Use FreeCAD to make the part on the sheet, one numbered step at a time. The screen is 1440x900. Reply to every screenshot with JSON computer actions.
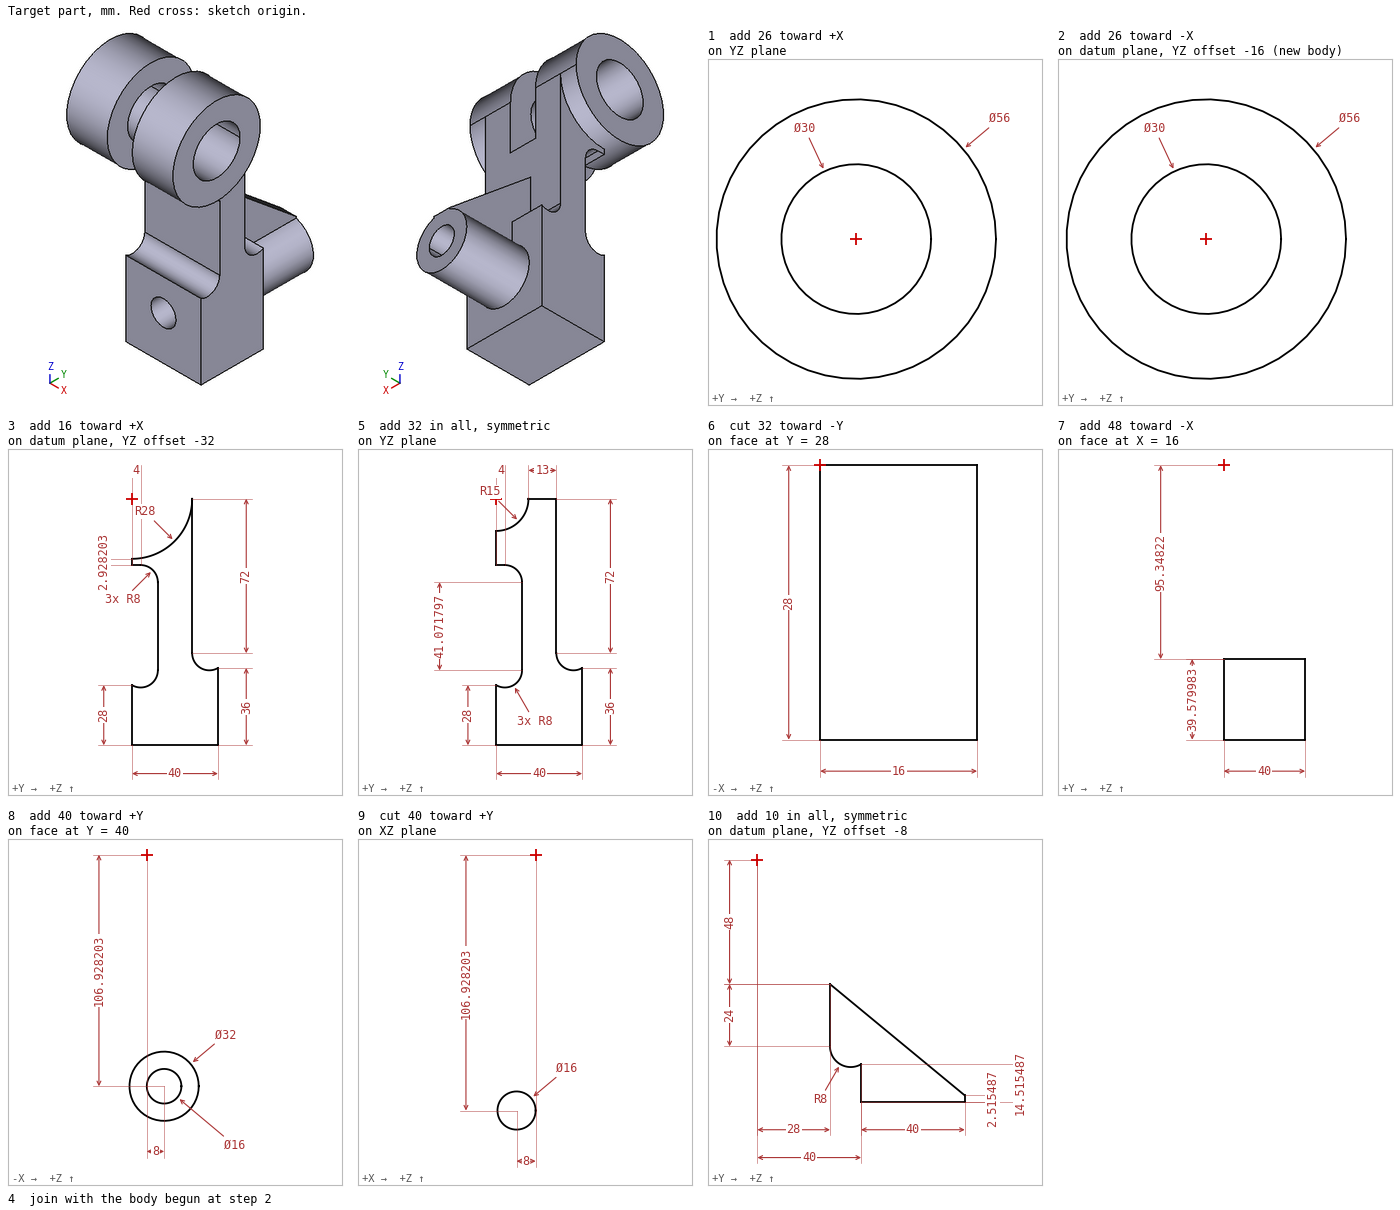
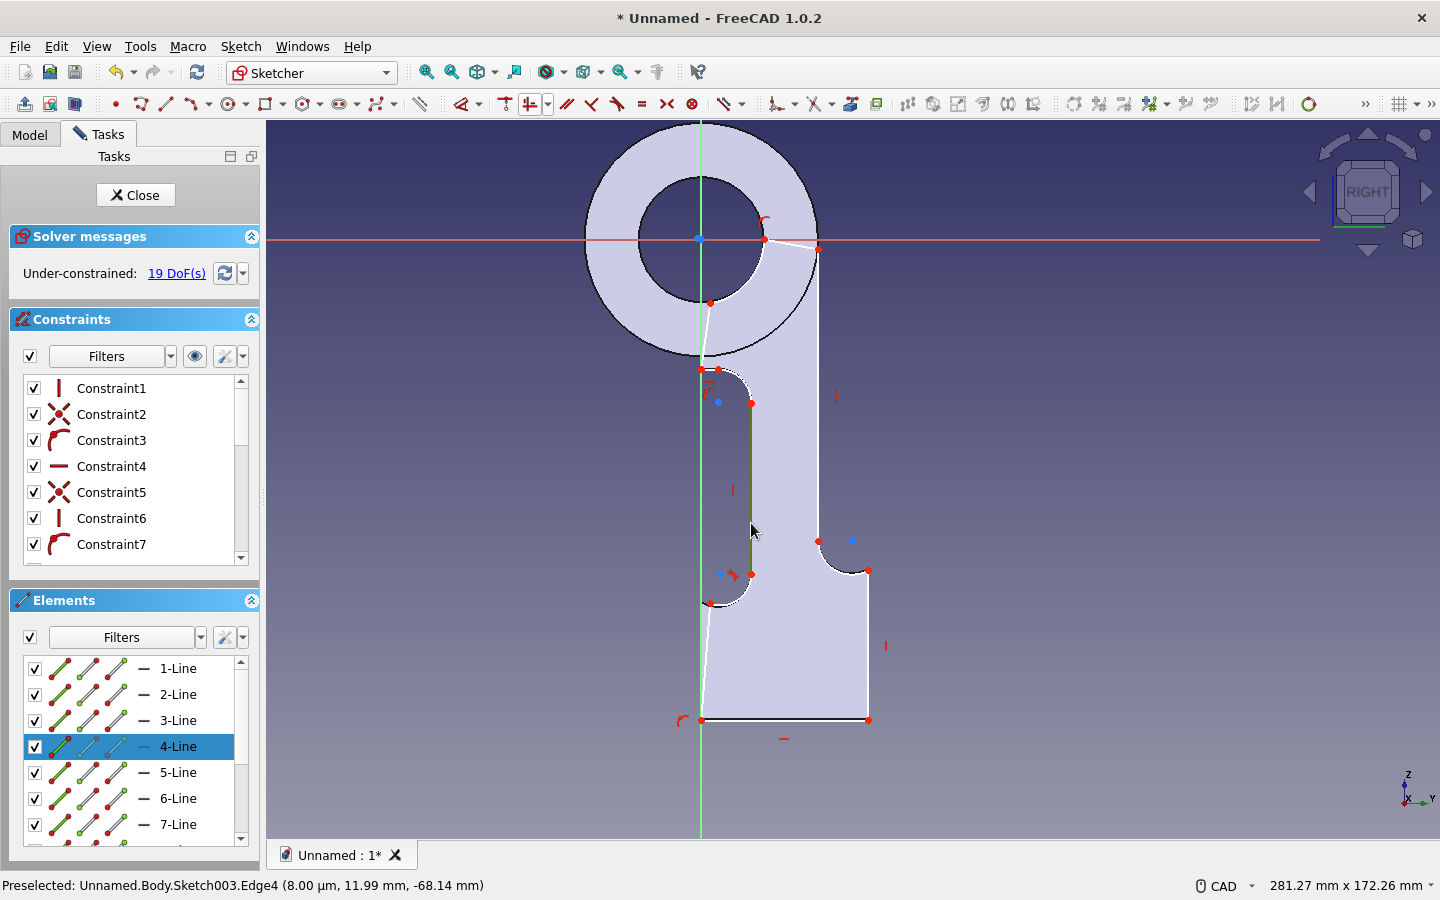
{"action": "left_click", "coordinate": [748, 388]}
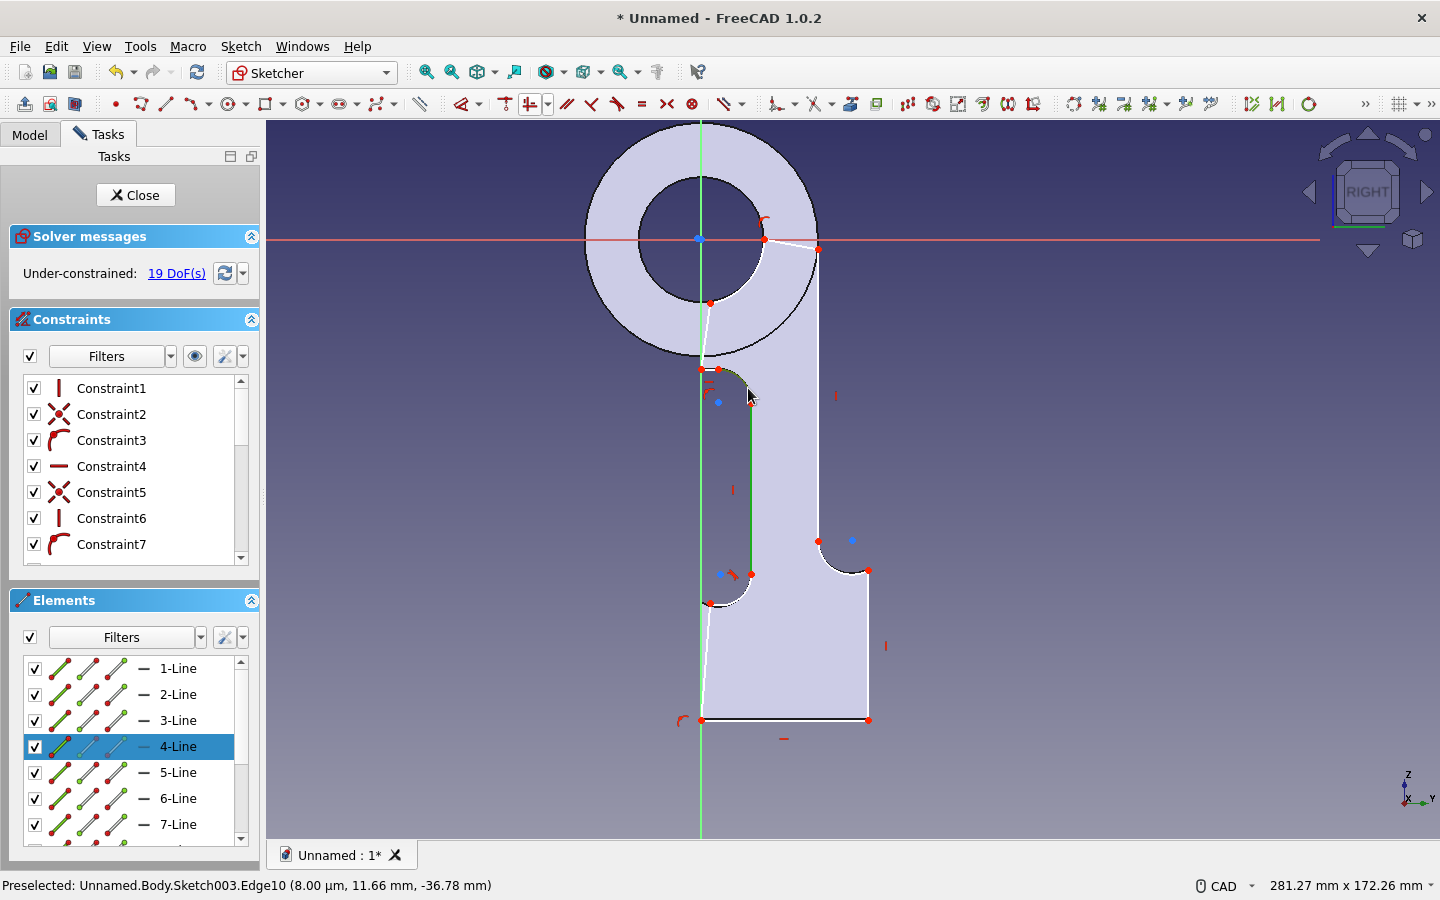
{"action": "key", "text": "t"}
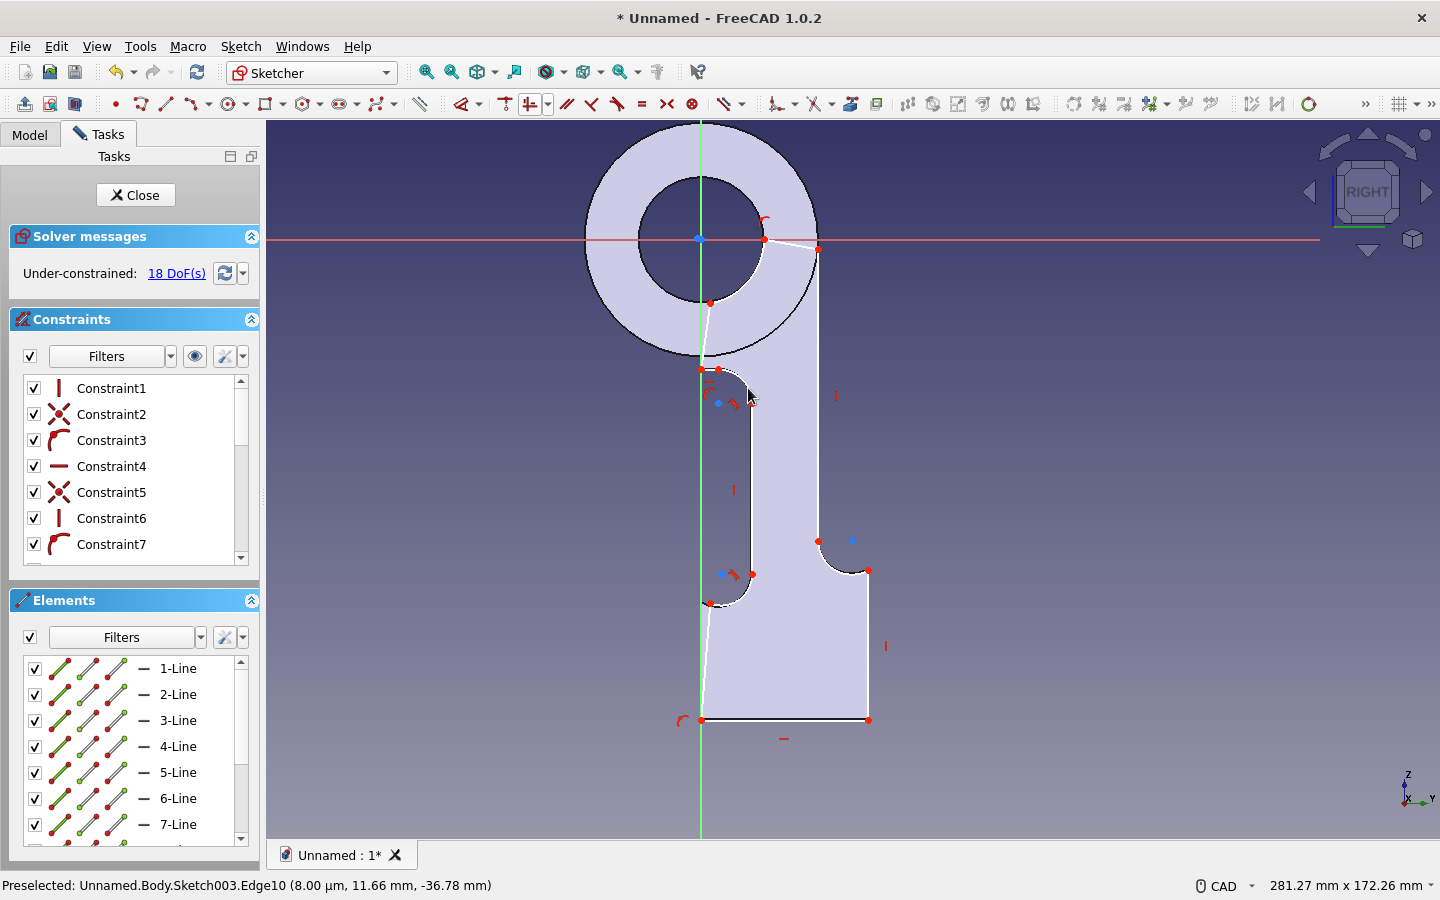
{"action": "scroll", "coordinate": [710, 370], "scroll_direction": "up", "scroll_amount": 3}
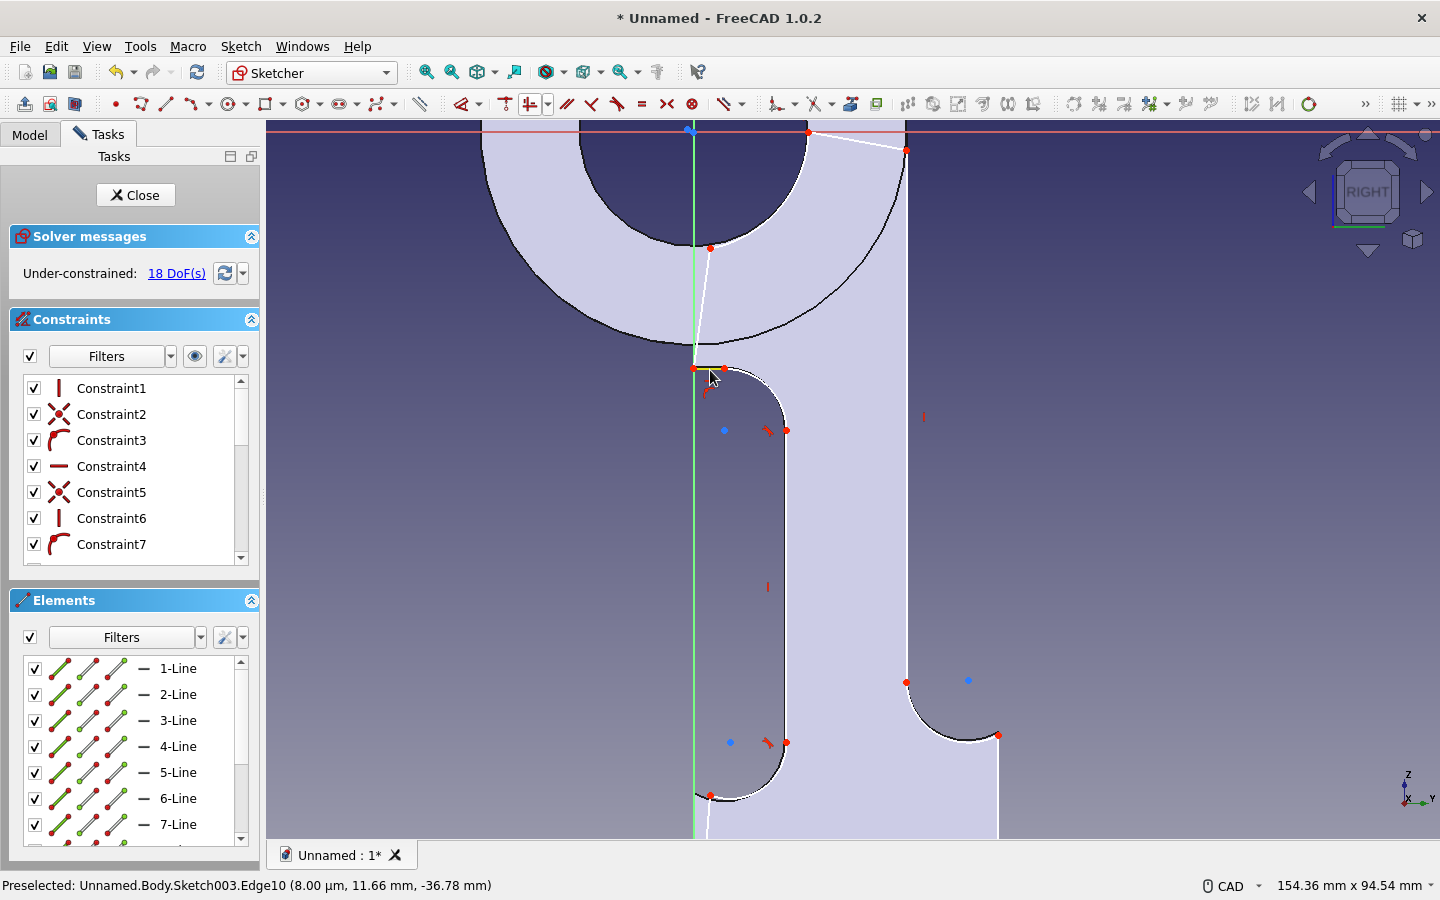
{"action": "left_click", "coordinate": [709, 369]}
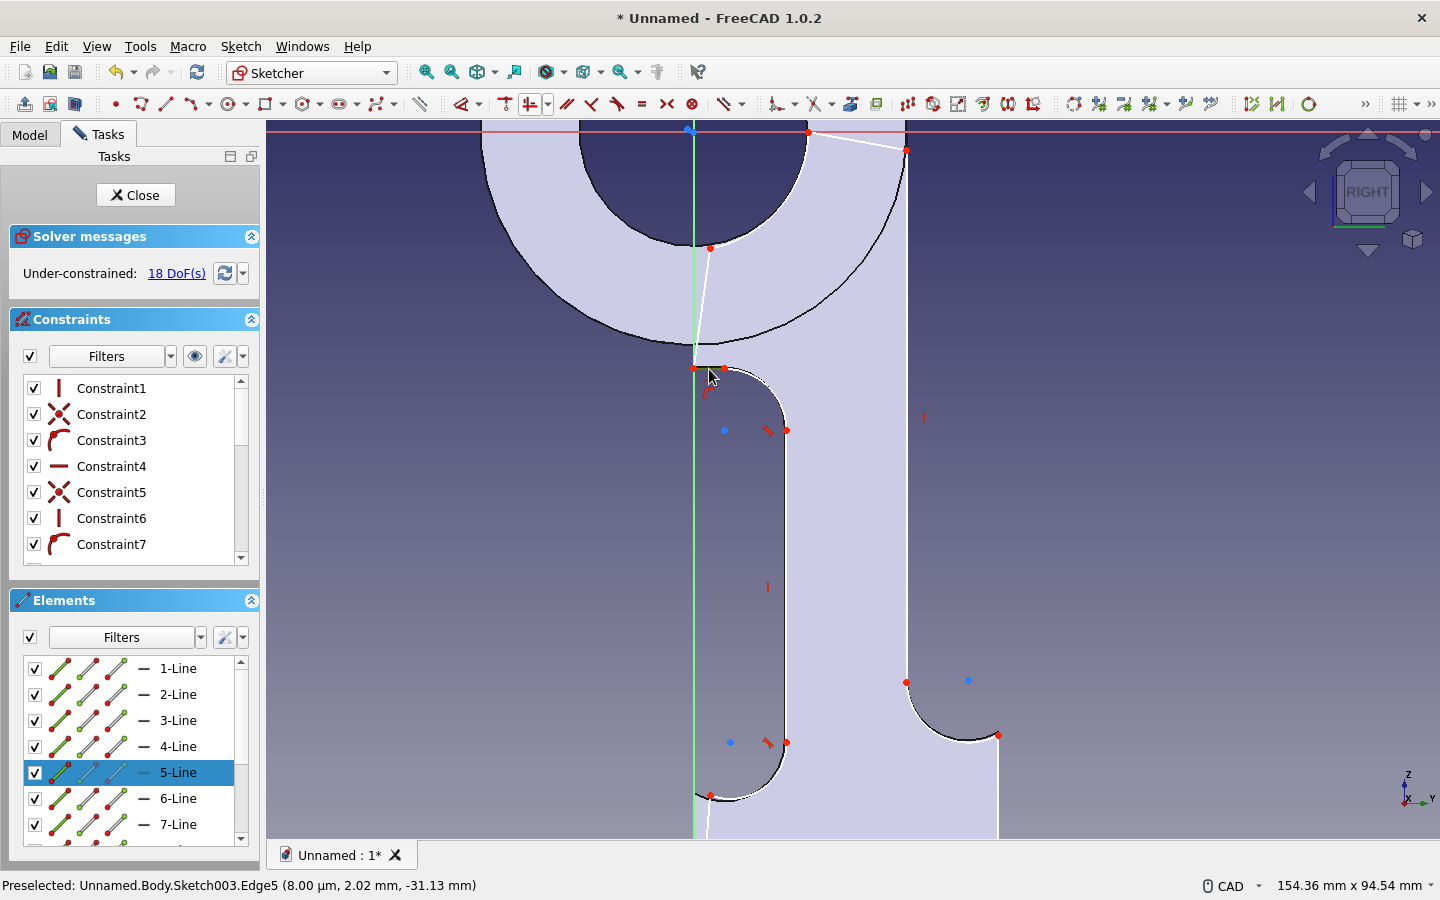
{"action": "left_click", "coordinate": [780, 403]}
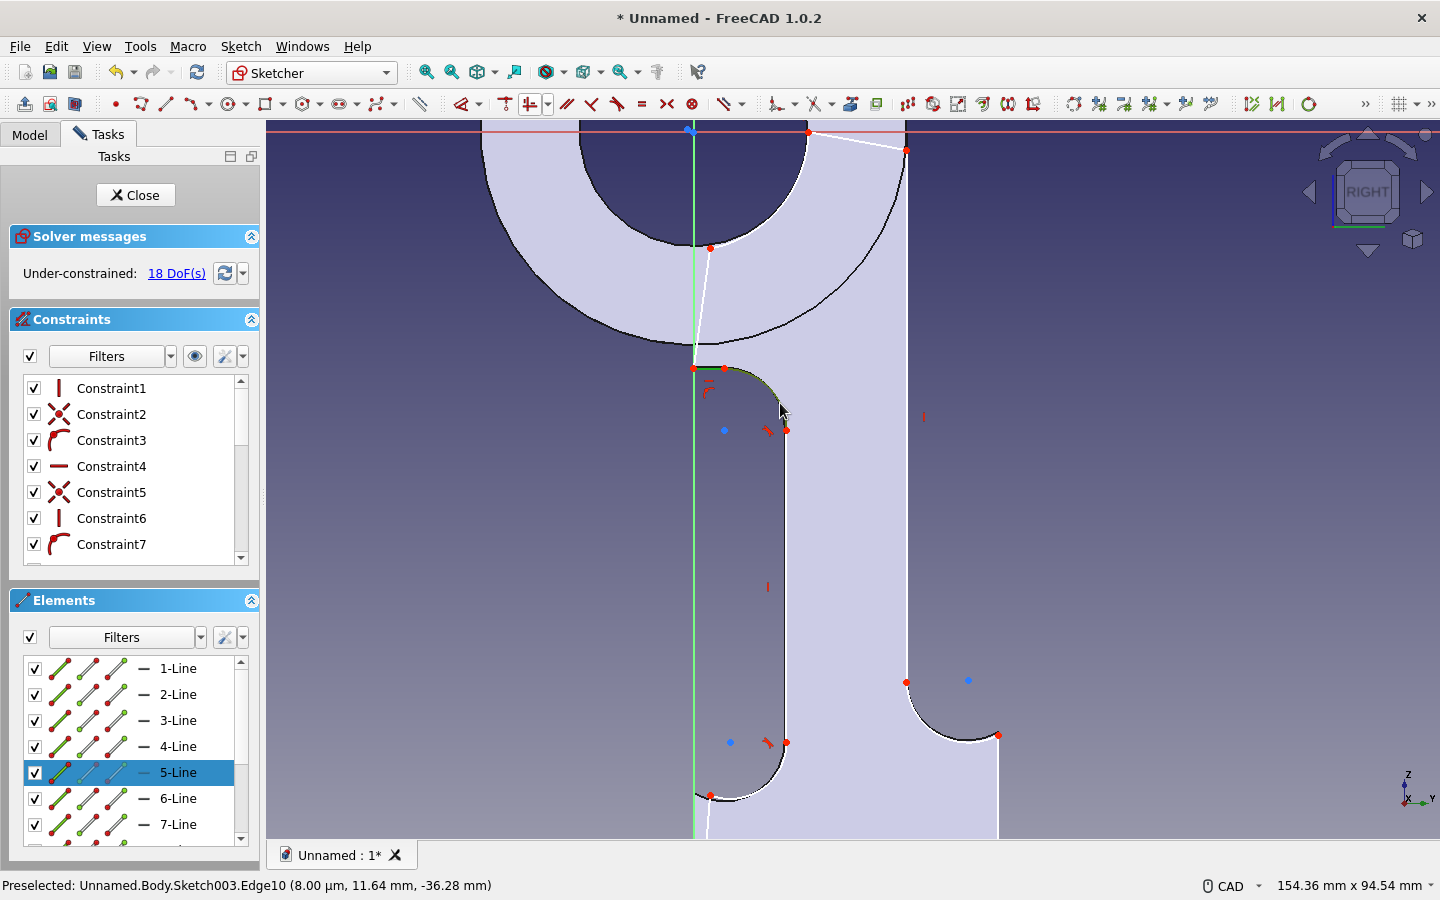
{"action": "key", "text": "t"}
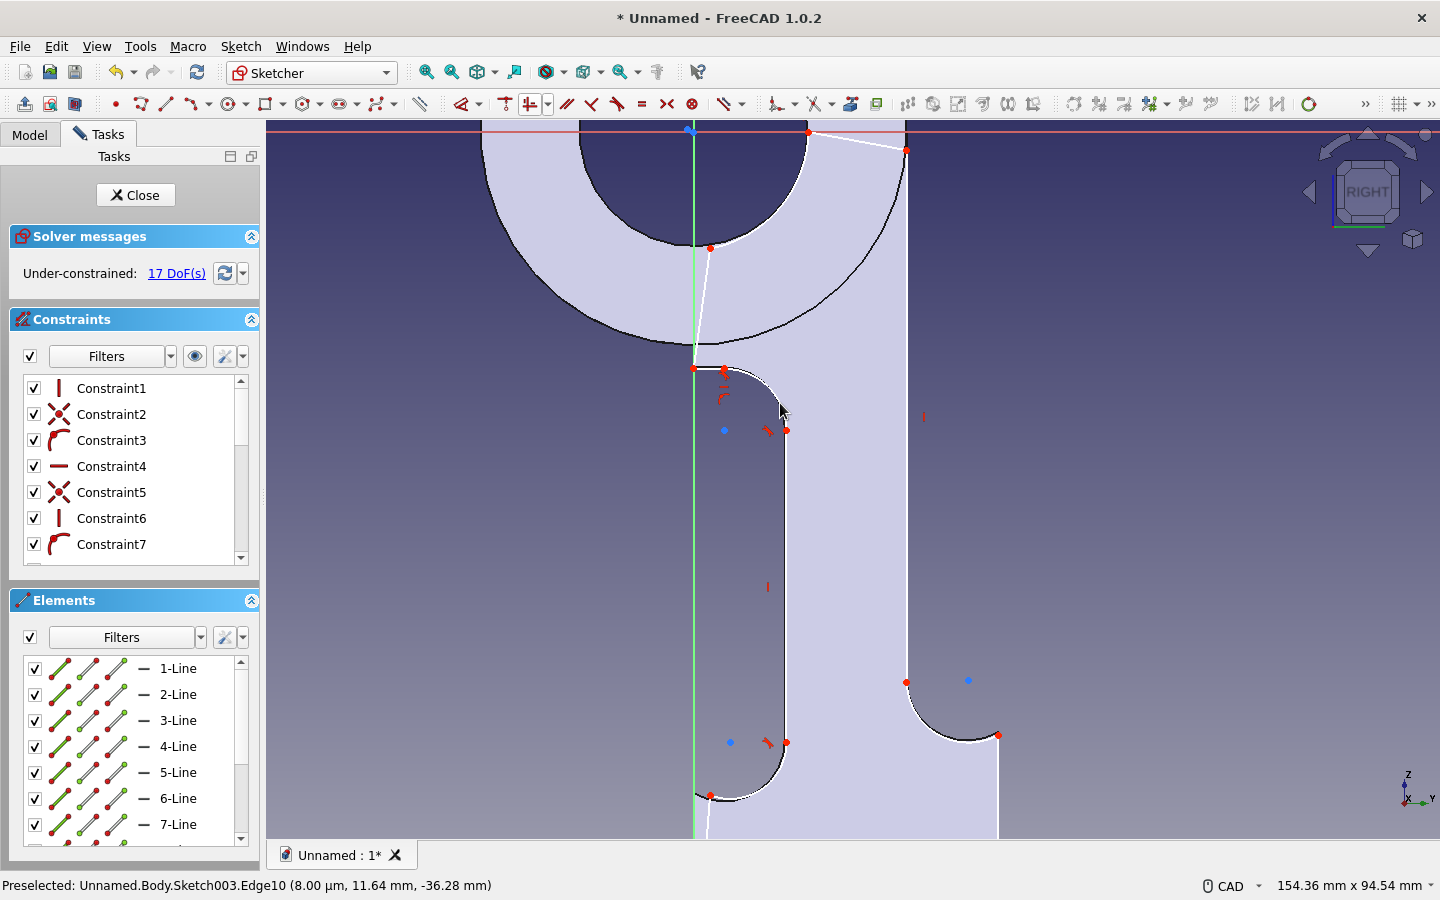
{"action": "left_click", "coordinate": [907, 310]}